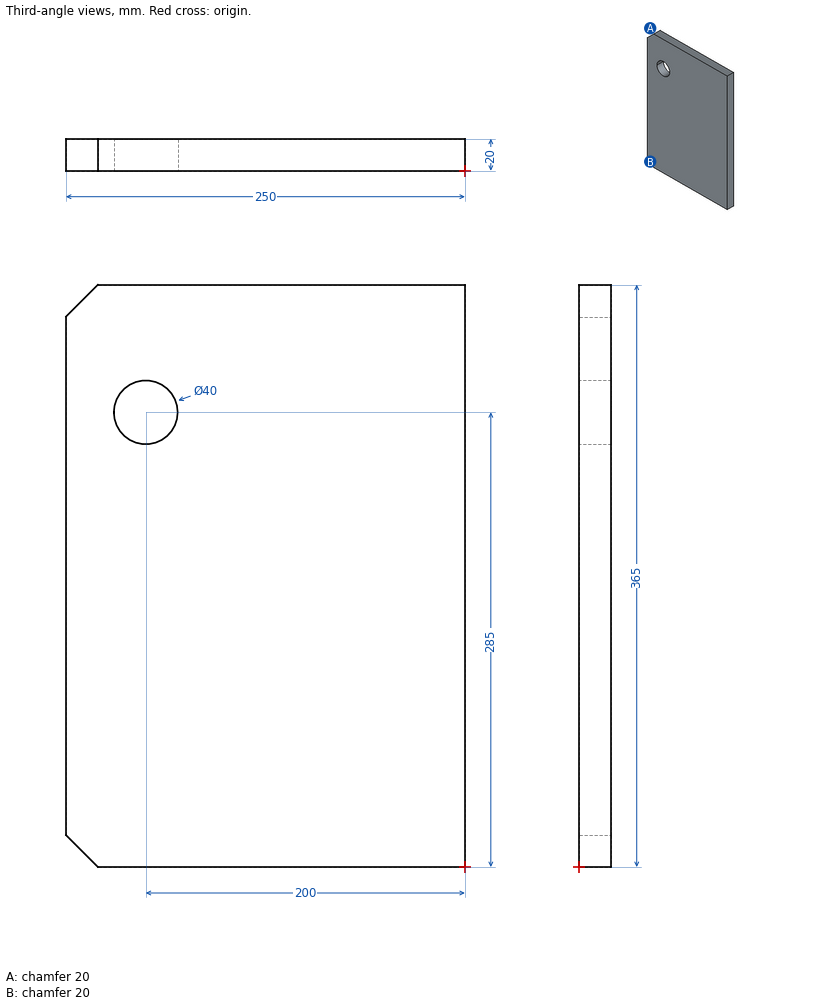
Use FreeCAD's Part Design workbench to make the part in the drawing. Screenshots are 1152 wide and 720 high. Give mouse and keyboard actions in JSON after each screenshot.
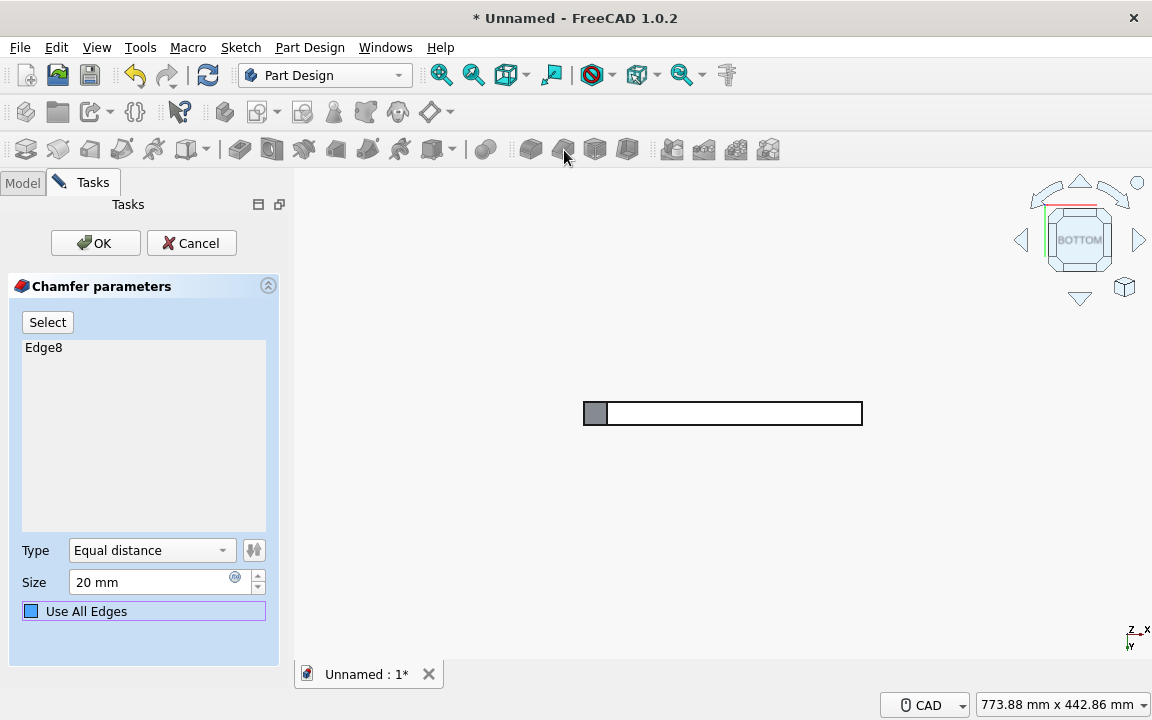
{"action": "left_click", "coordinate": [96, 243]}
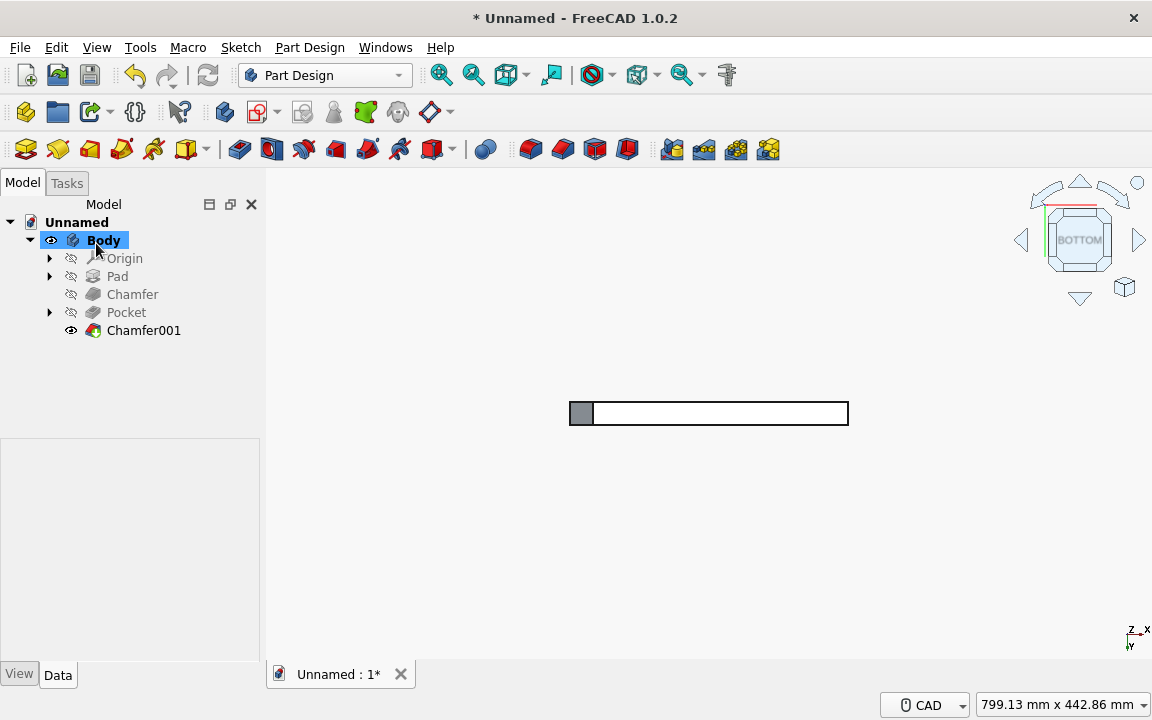
{"action": "key", "text": "0"}